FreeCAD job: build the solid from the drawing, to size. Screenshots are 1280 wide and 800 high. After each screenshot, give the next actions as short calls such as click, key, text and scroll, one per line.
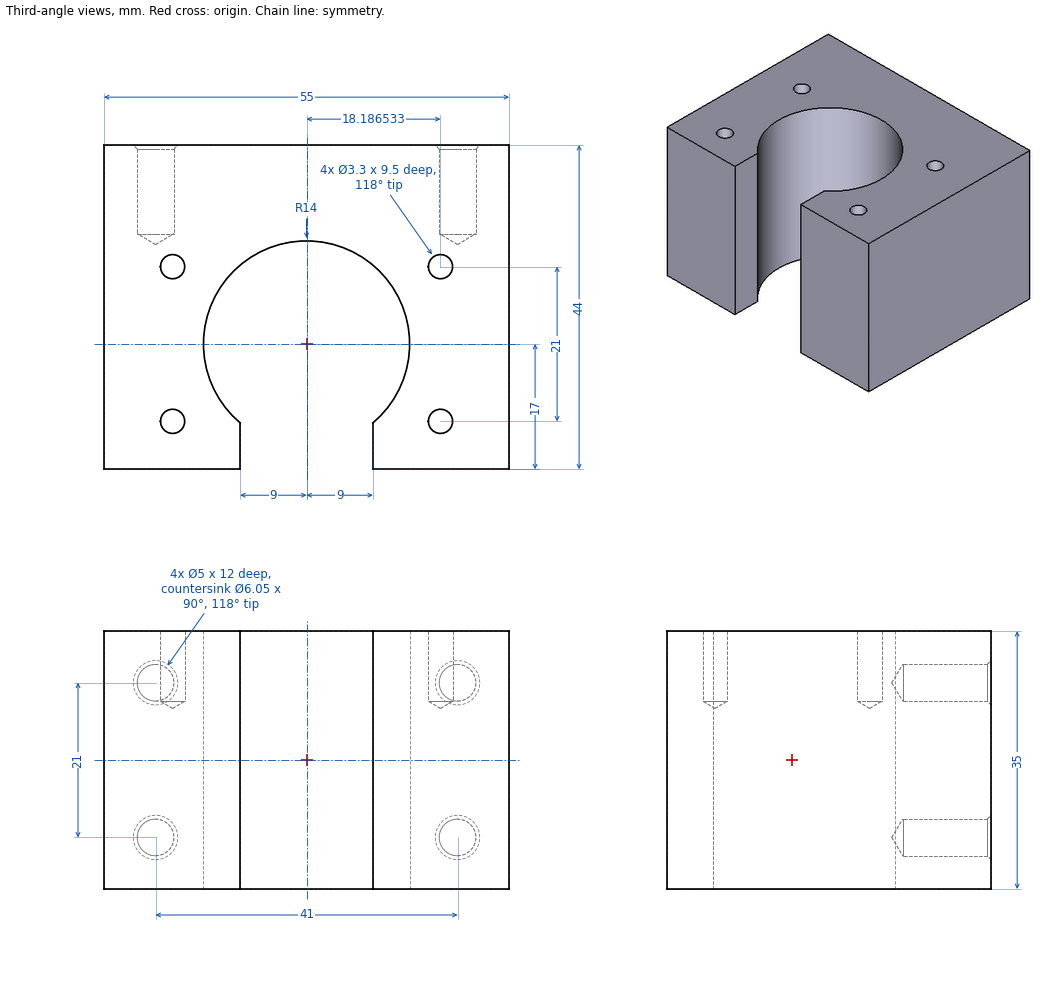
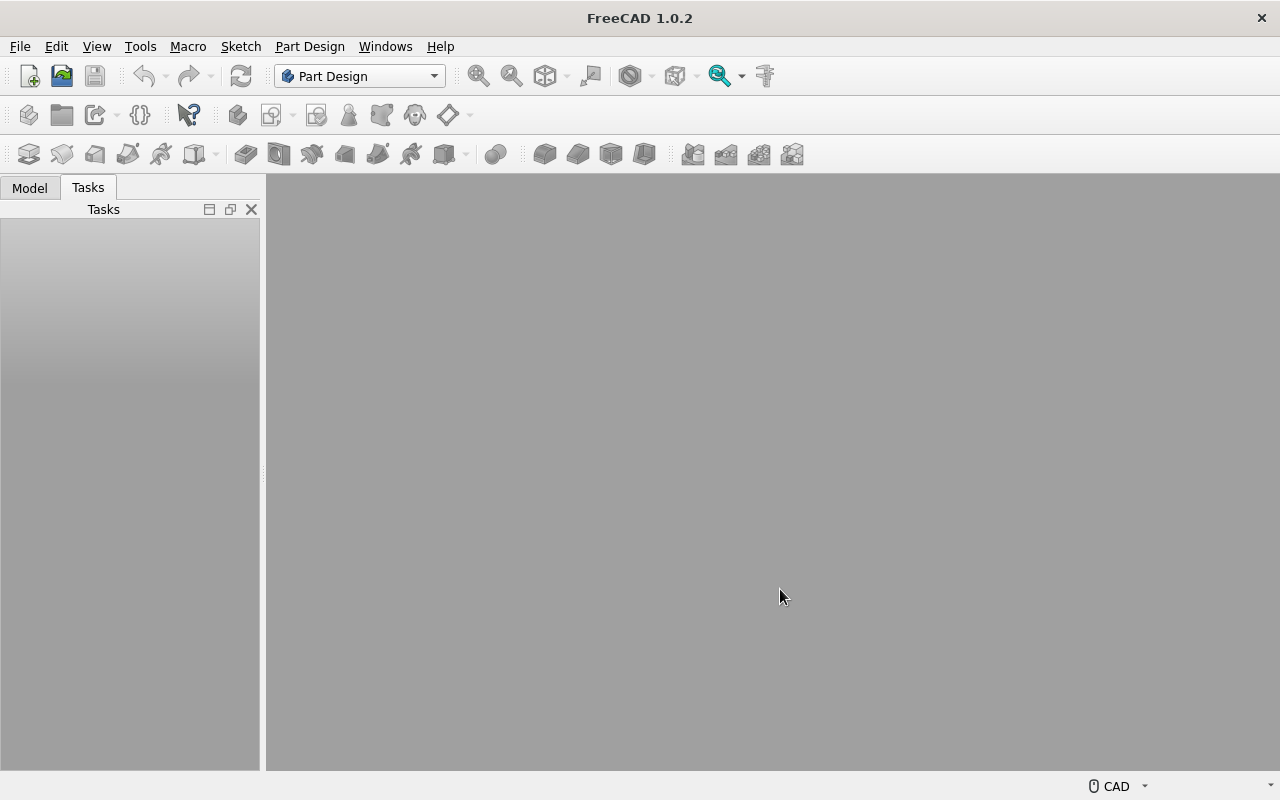
click(29, 76)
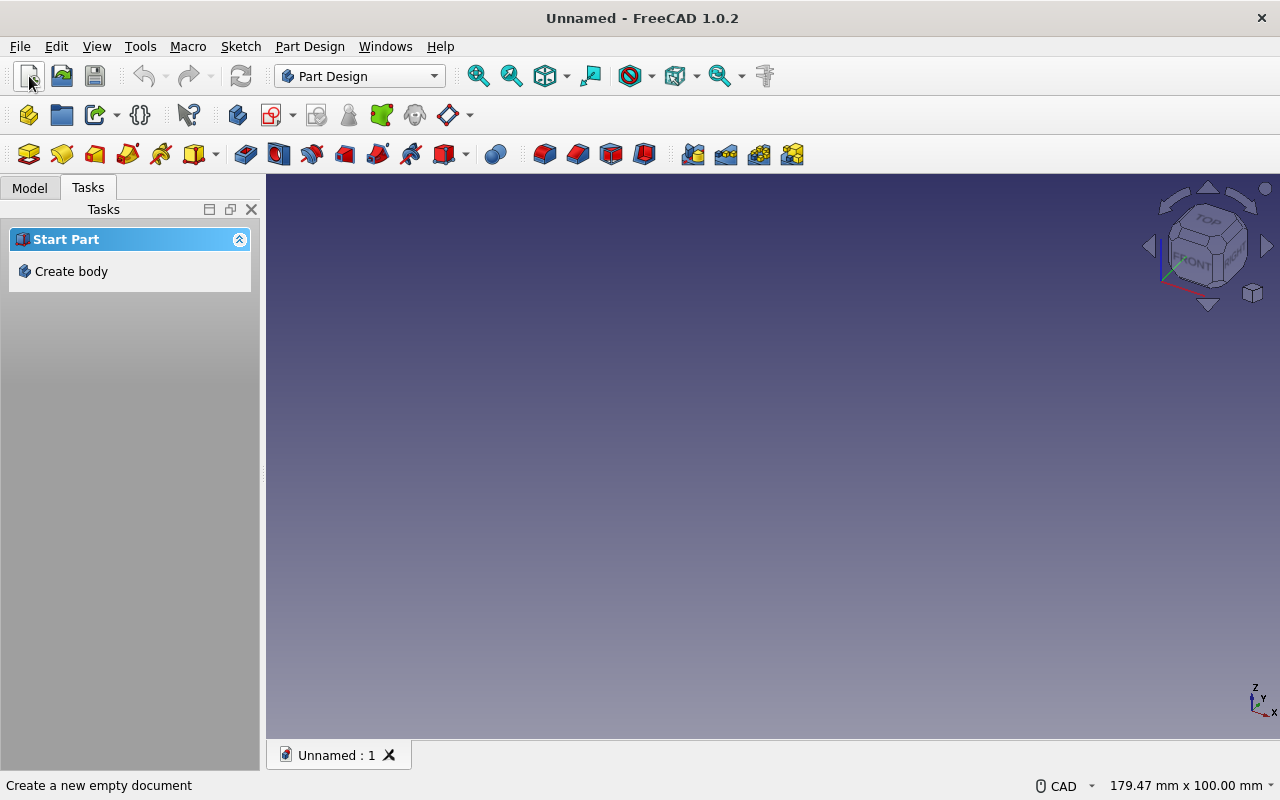
click(270, 116)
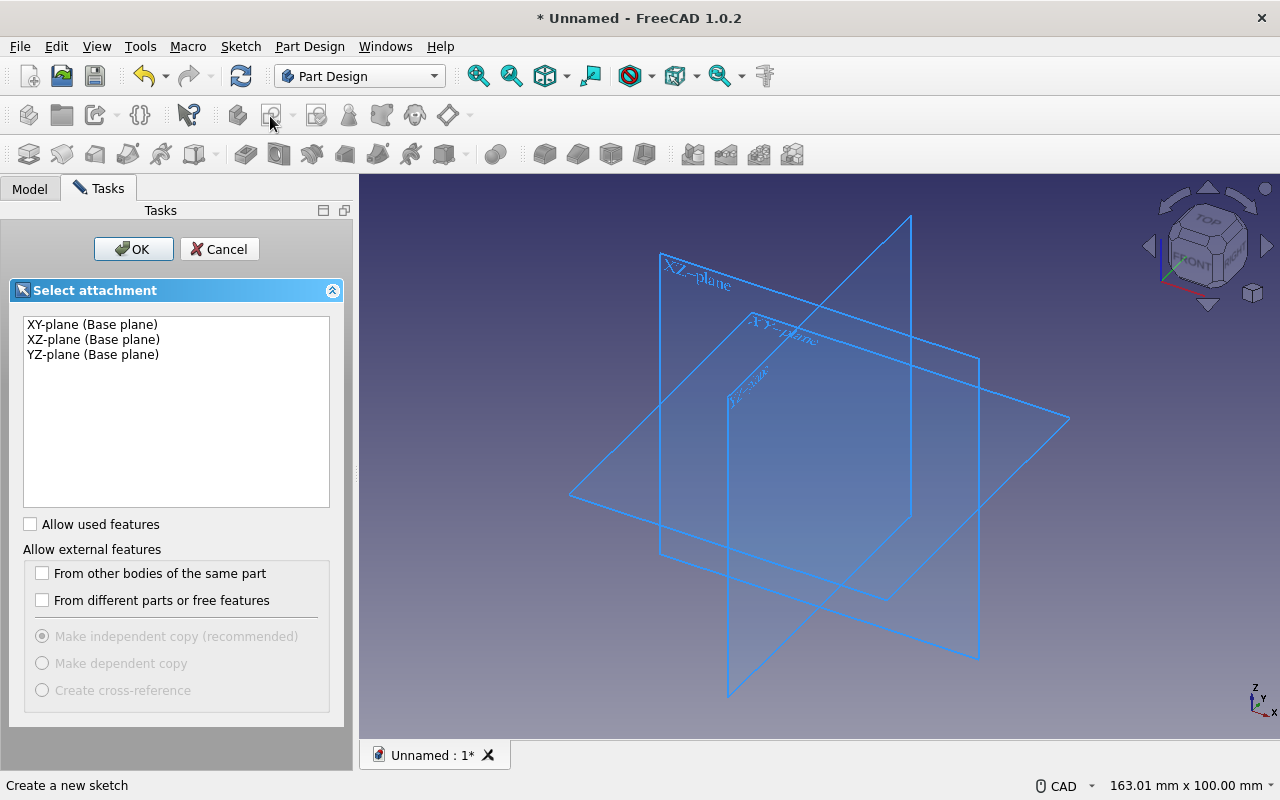
click(84, 324)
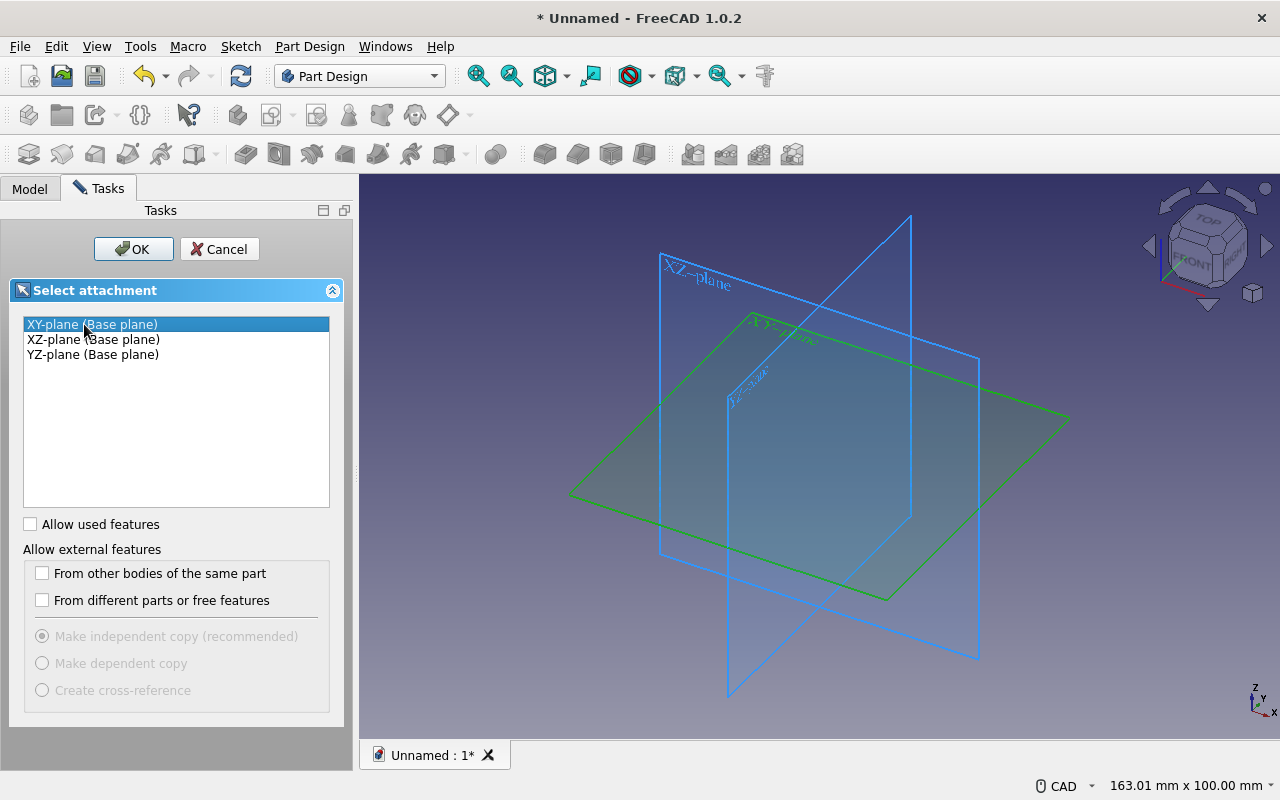
click(134, 249)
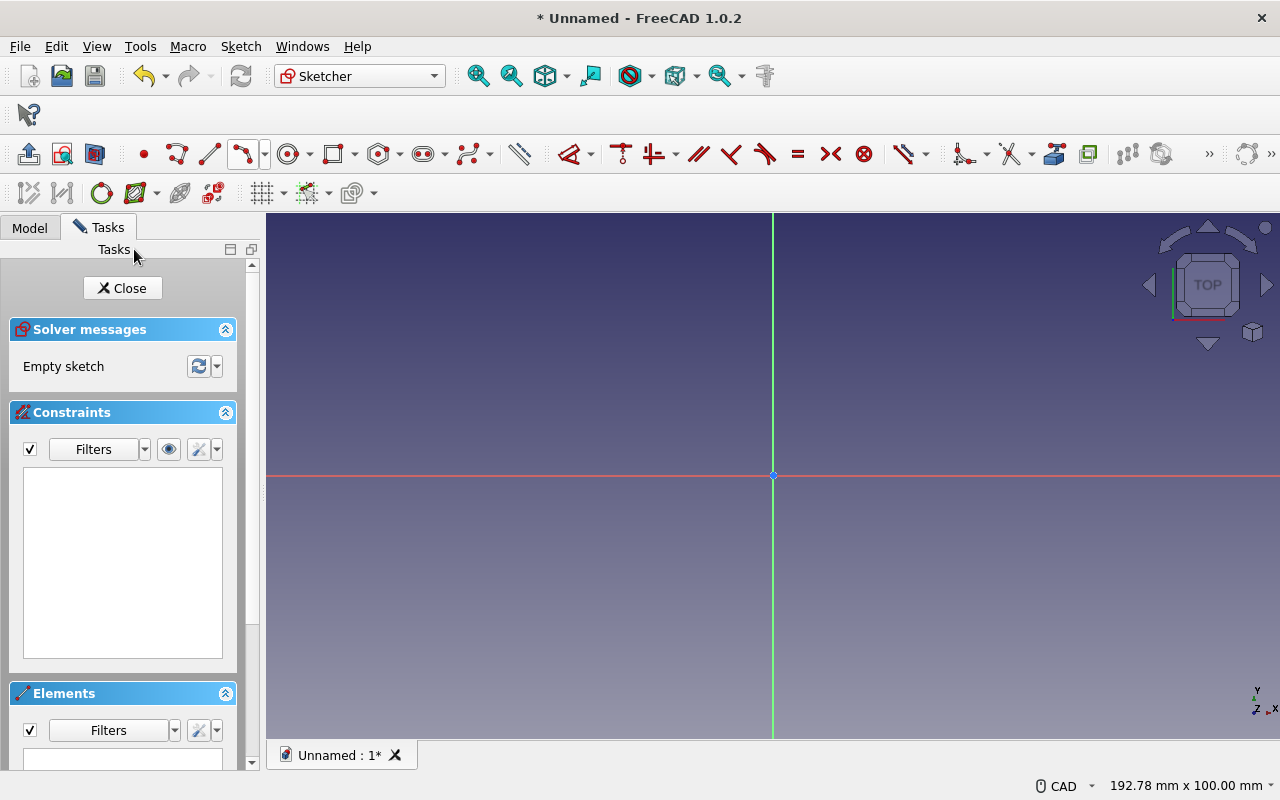
scroll(912, 396, up, 2)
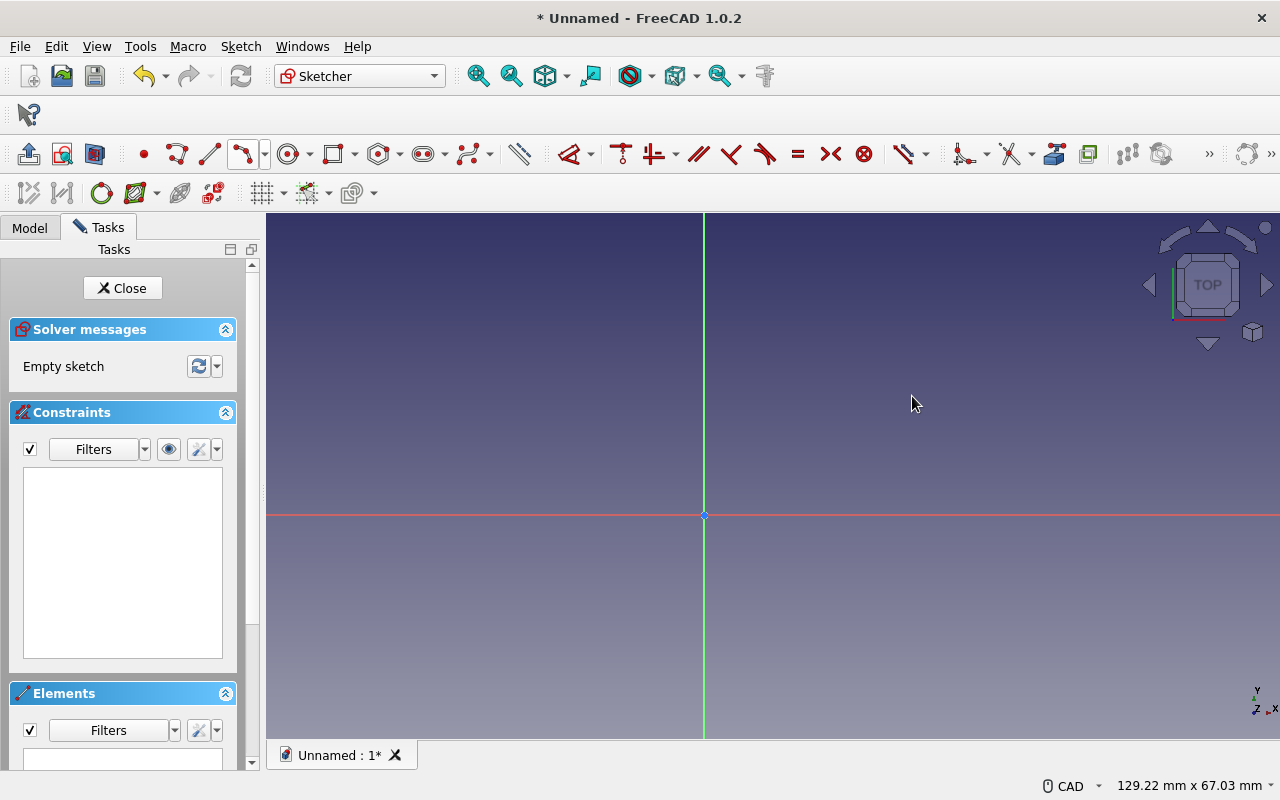
click(177, 154)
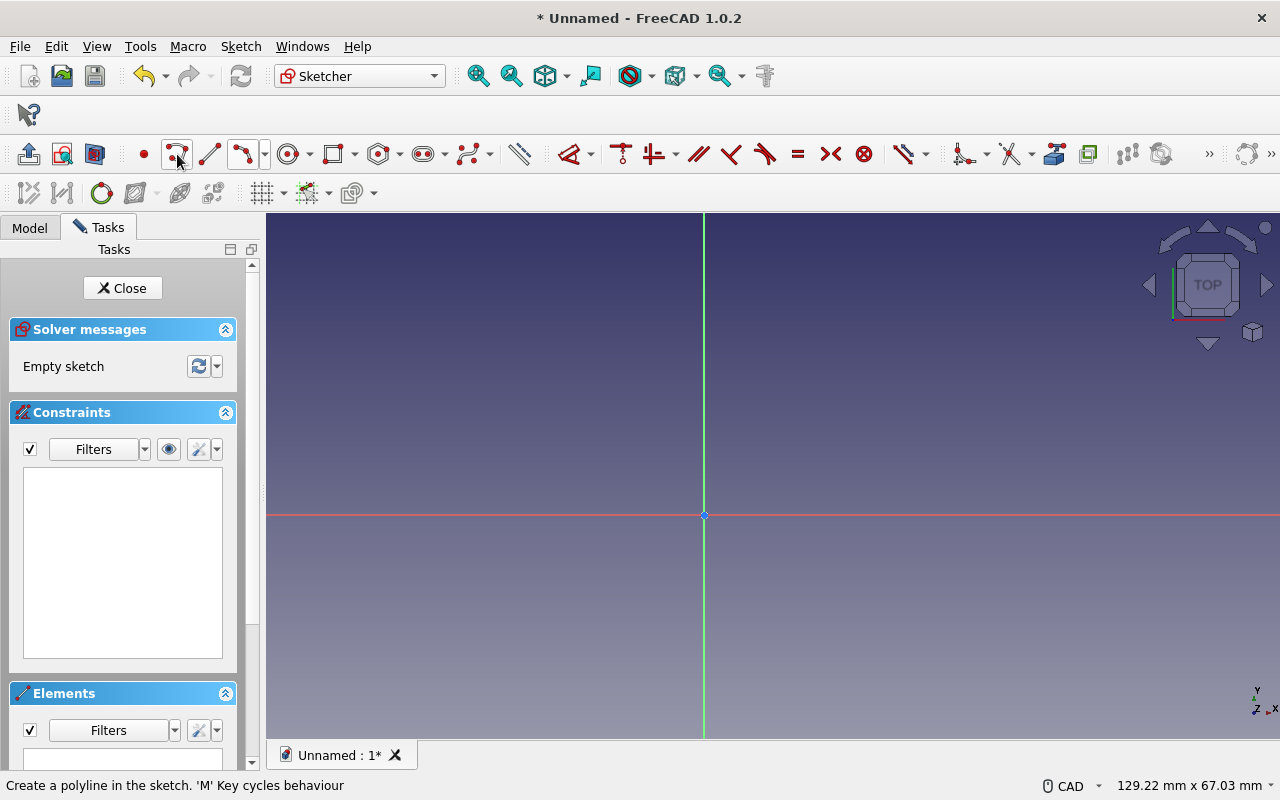
click(775, 599)
click(775, 649)
click(920, 649)
click(920, 303)
click(489, 303)
click(489, 649)
click(634, 649)
click(634, 599)
right_click(634, 599)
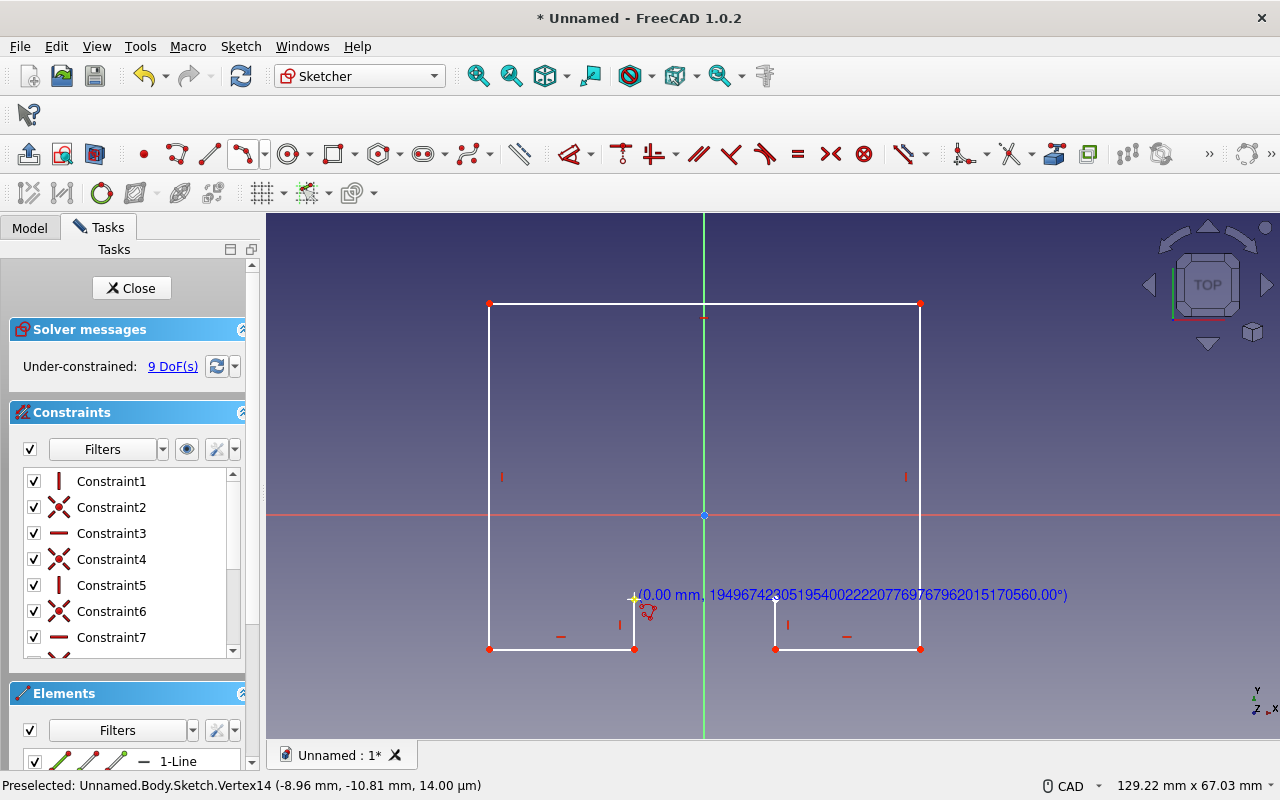
click(242, 154)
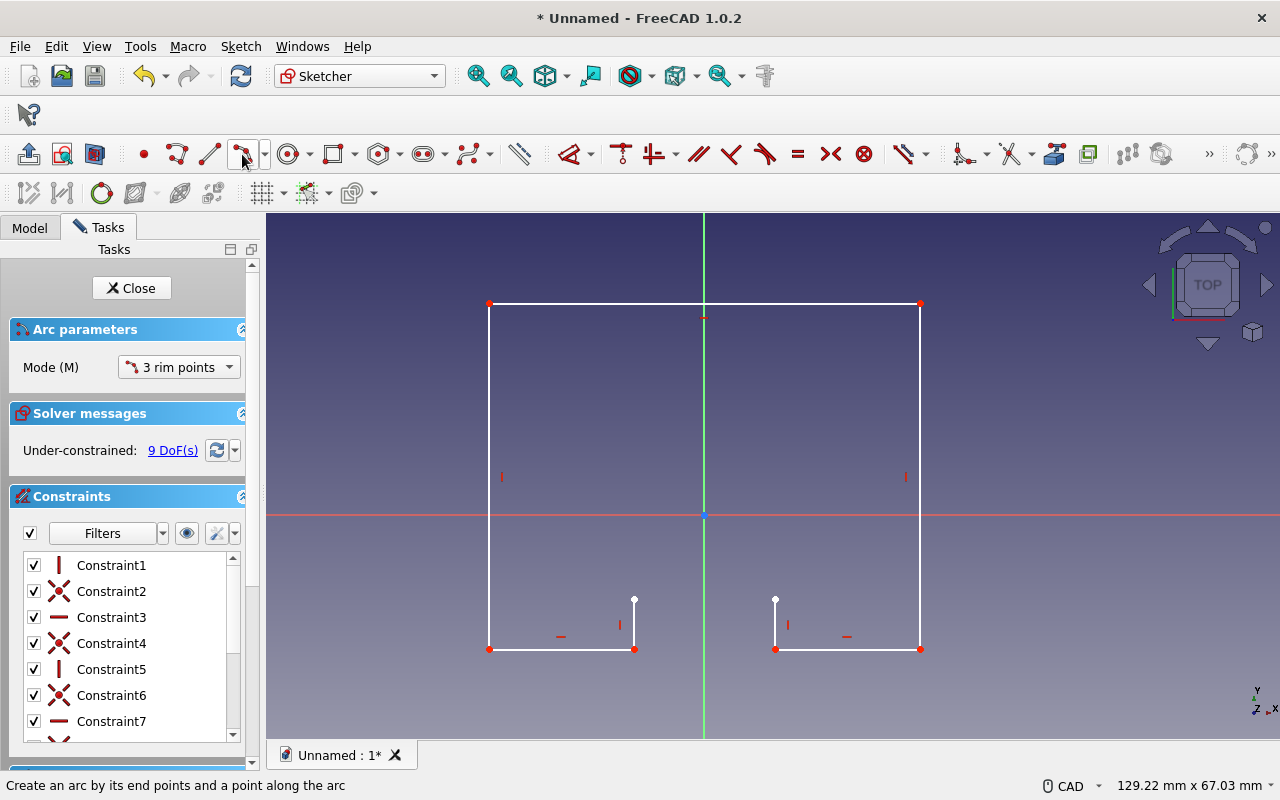
click(634, 600)
click(775, 600)
click(756, 418)
key(Escape)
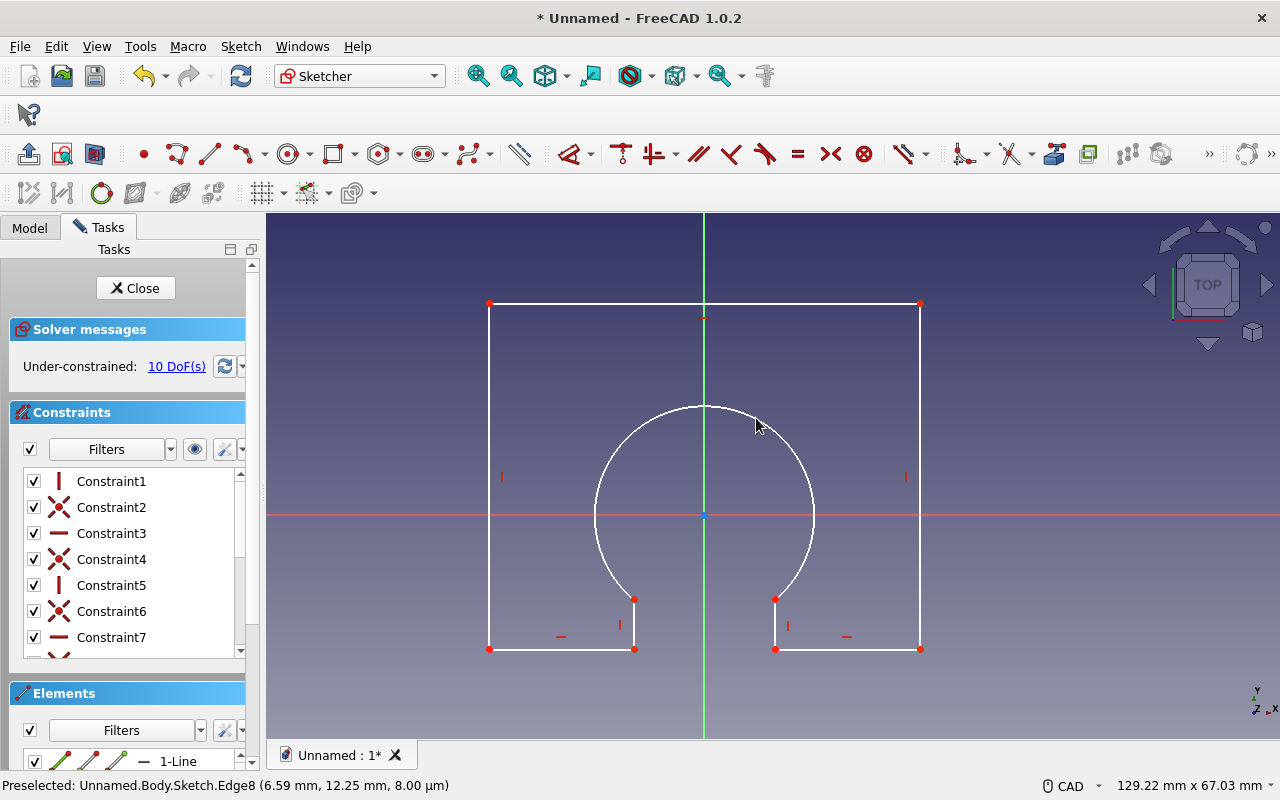
drag(694, 505, 714, 526)